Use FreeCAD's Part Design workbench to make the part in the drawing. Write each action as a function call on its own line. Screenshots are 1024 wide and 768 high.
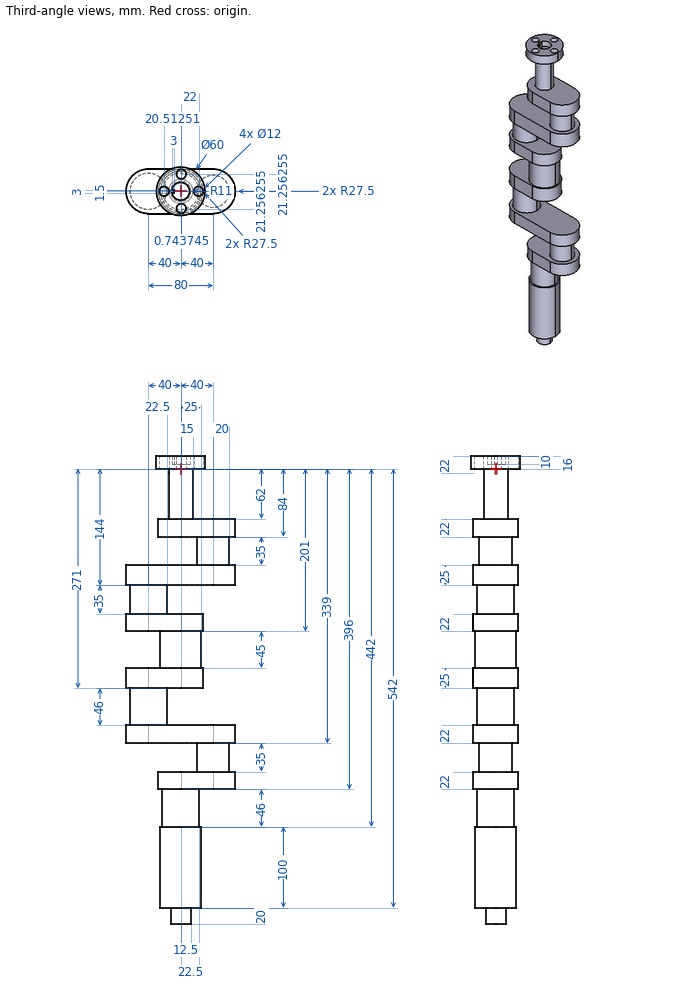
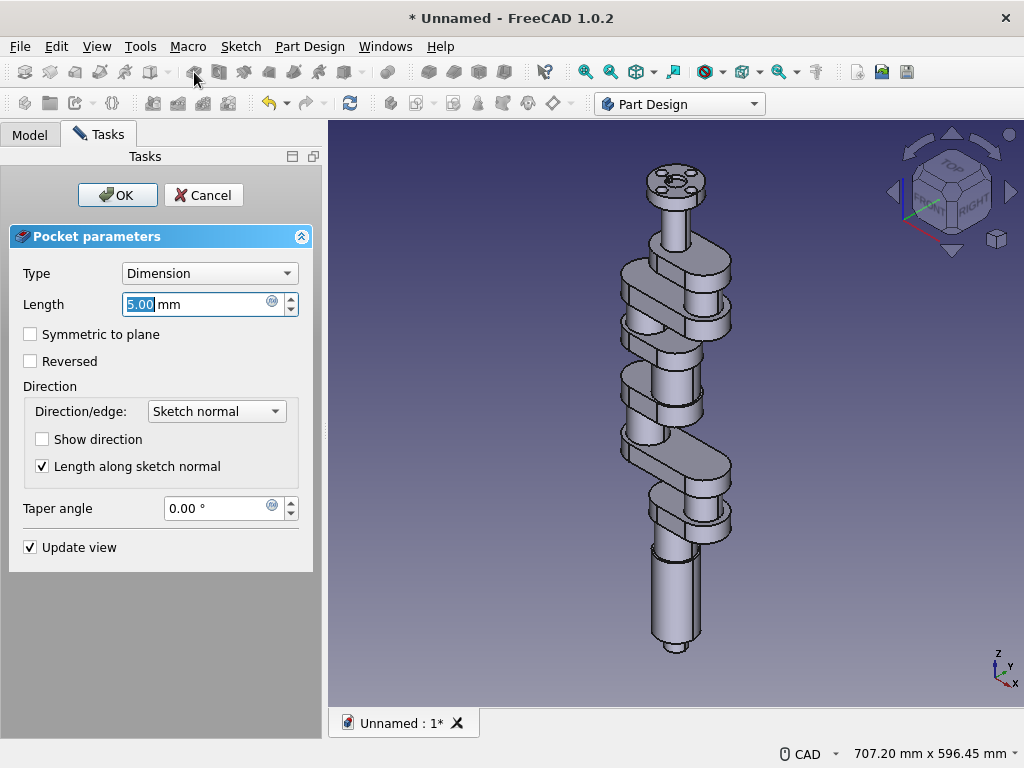
text(10)
key(Tab)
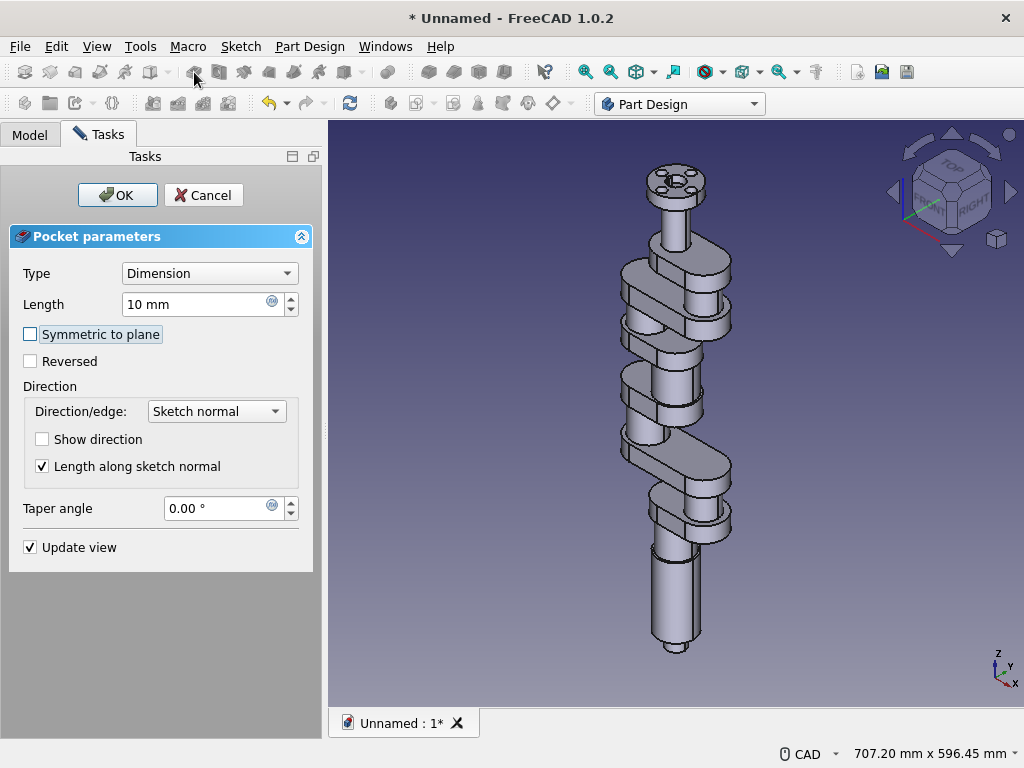
click(118, 195)